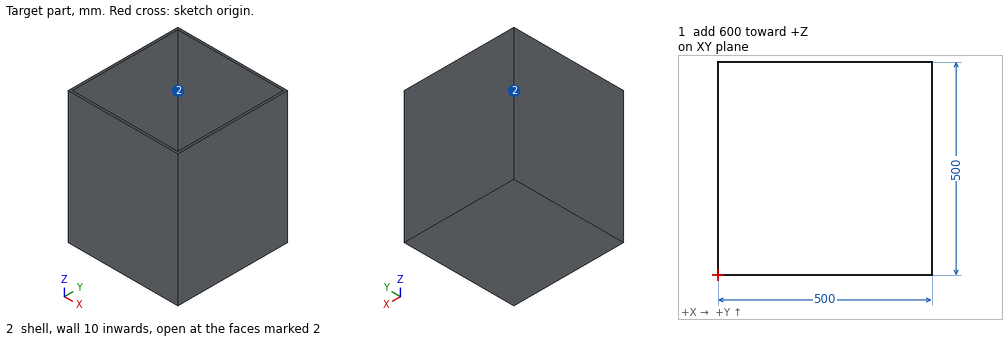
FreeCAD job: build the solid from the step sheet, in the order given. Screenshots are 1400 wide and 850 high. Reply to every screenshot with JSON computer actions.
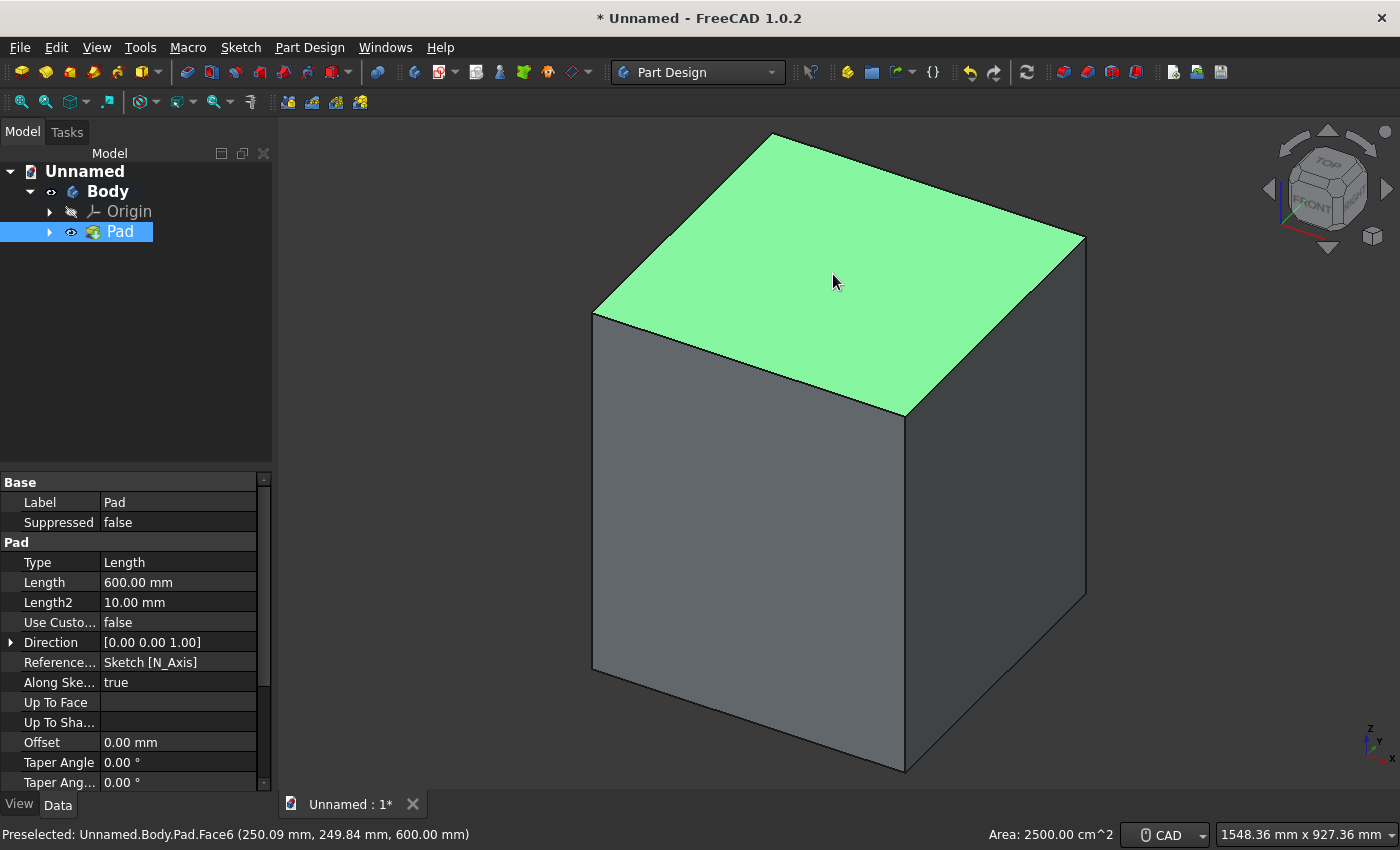
{"action": "left_click", "coordinate": [1136, 72]}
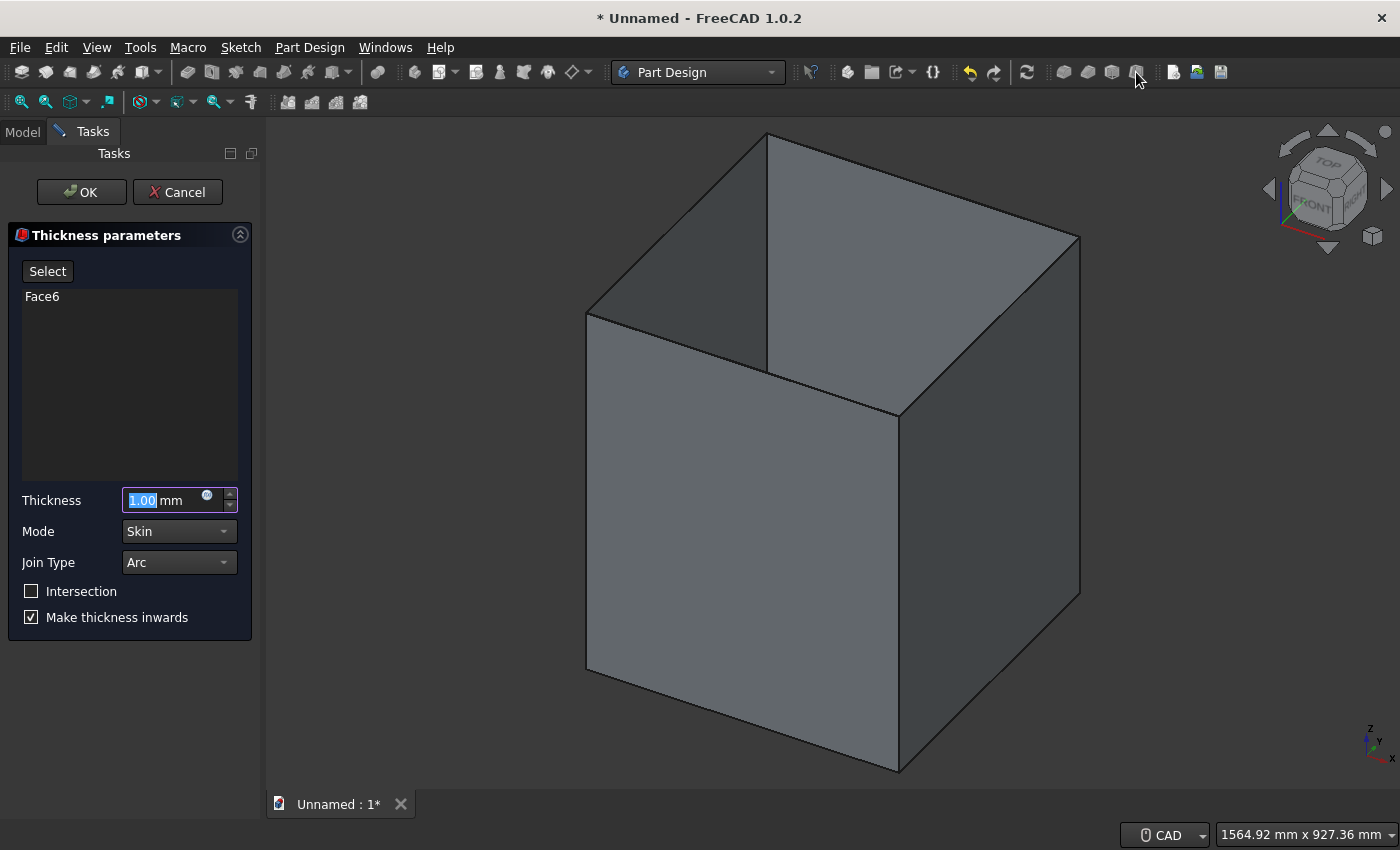
{"action": "type", "text": "10"}
{"action": "key", "text": "Tab"}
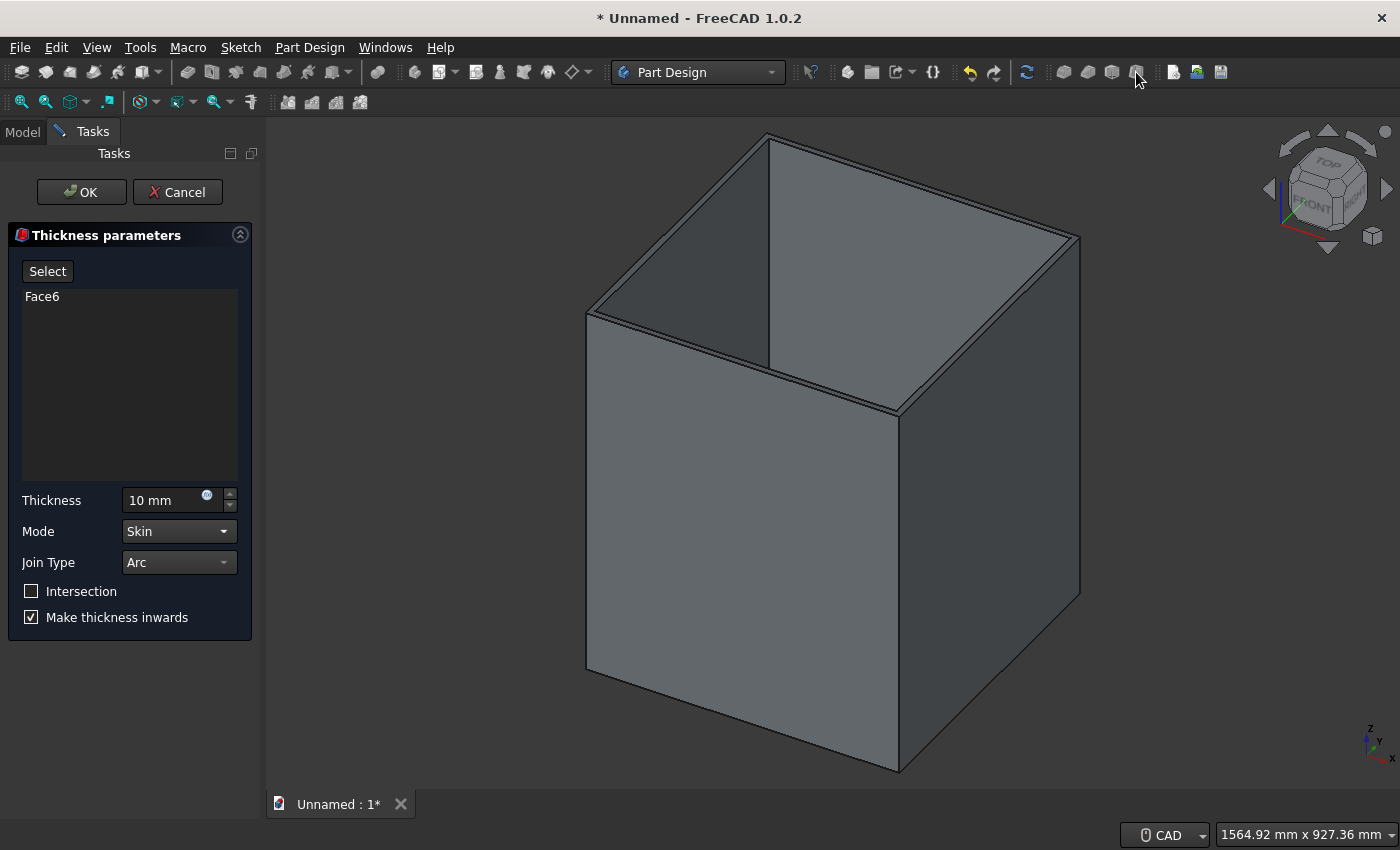
{"action": "left_click", "coordinate": [180, 562]}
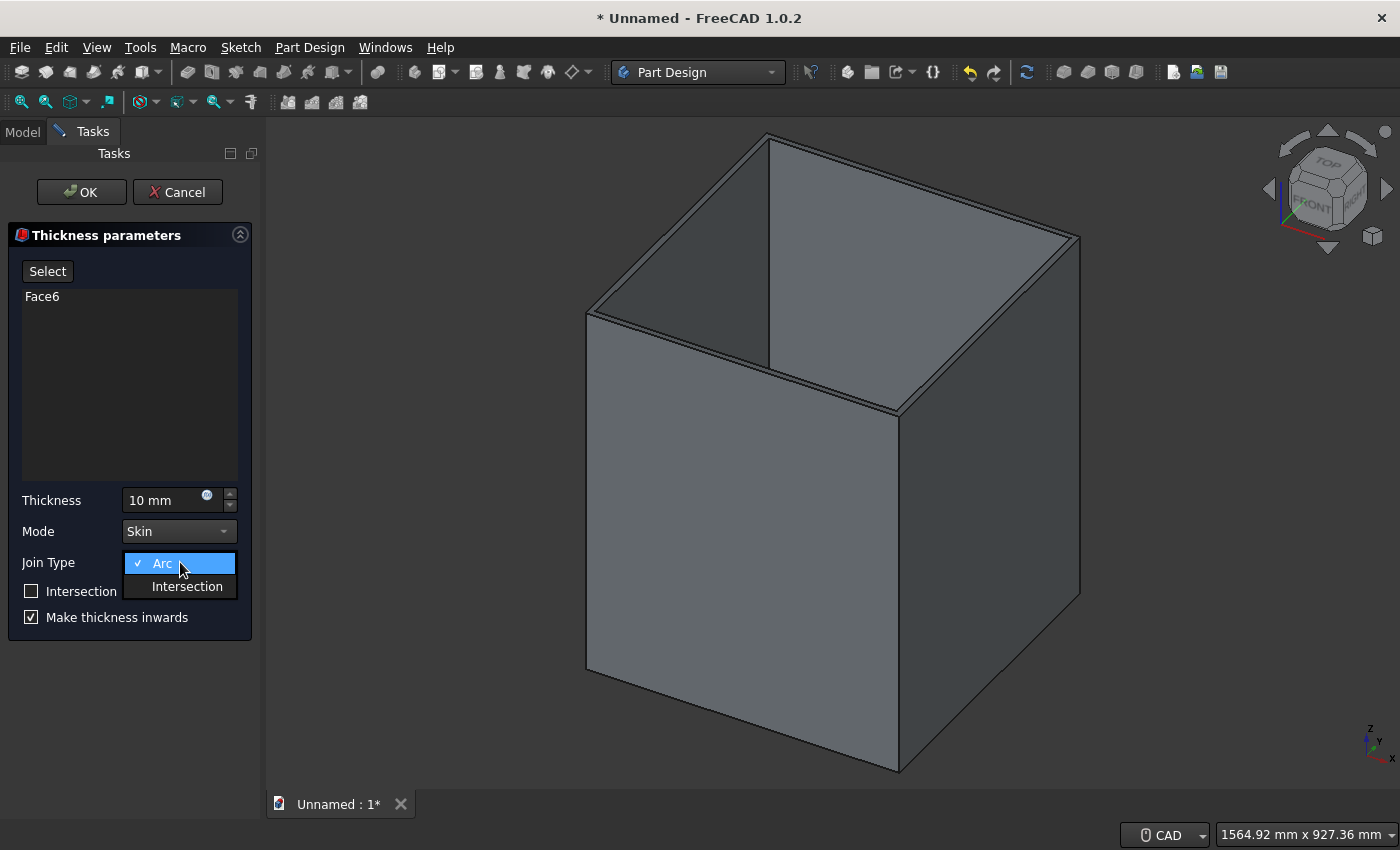
{"action": "left_click", "coordinate": [179, 586]}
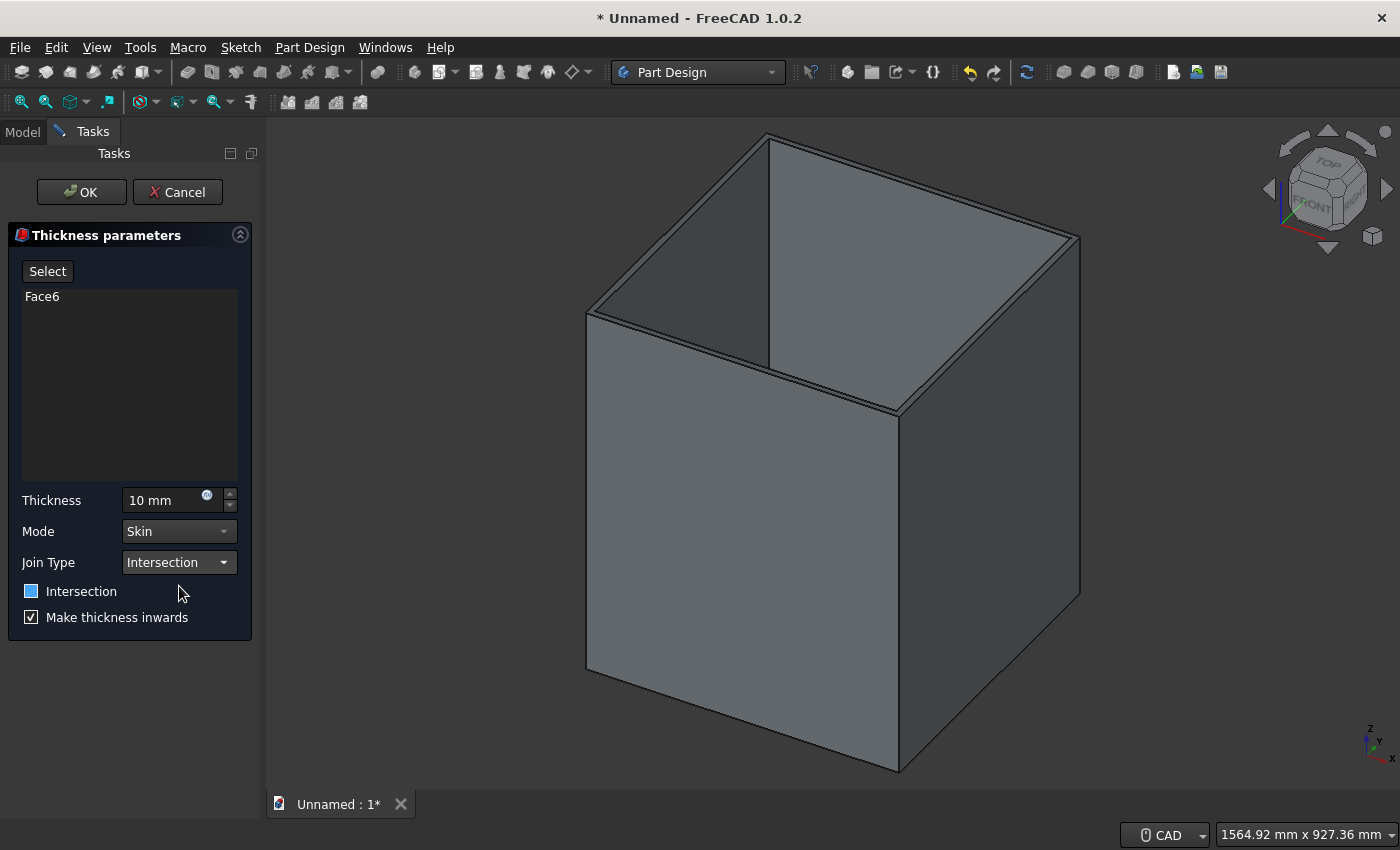
{"action": "left_click", "coordinate": [82, 192]}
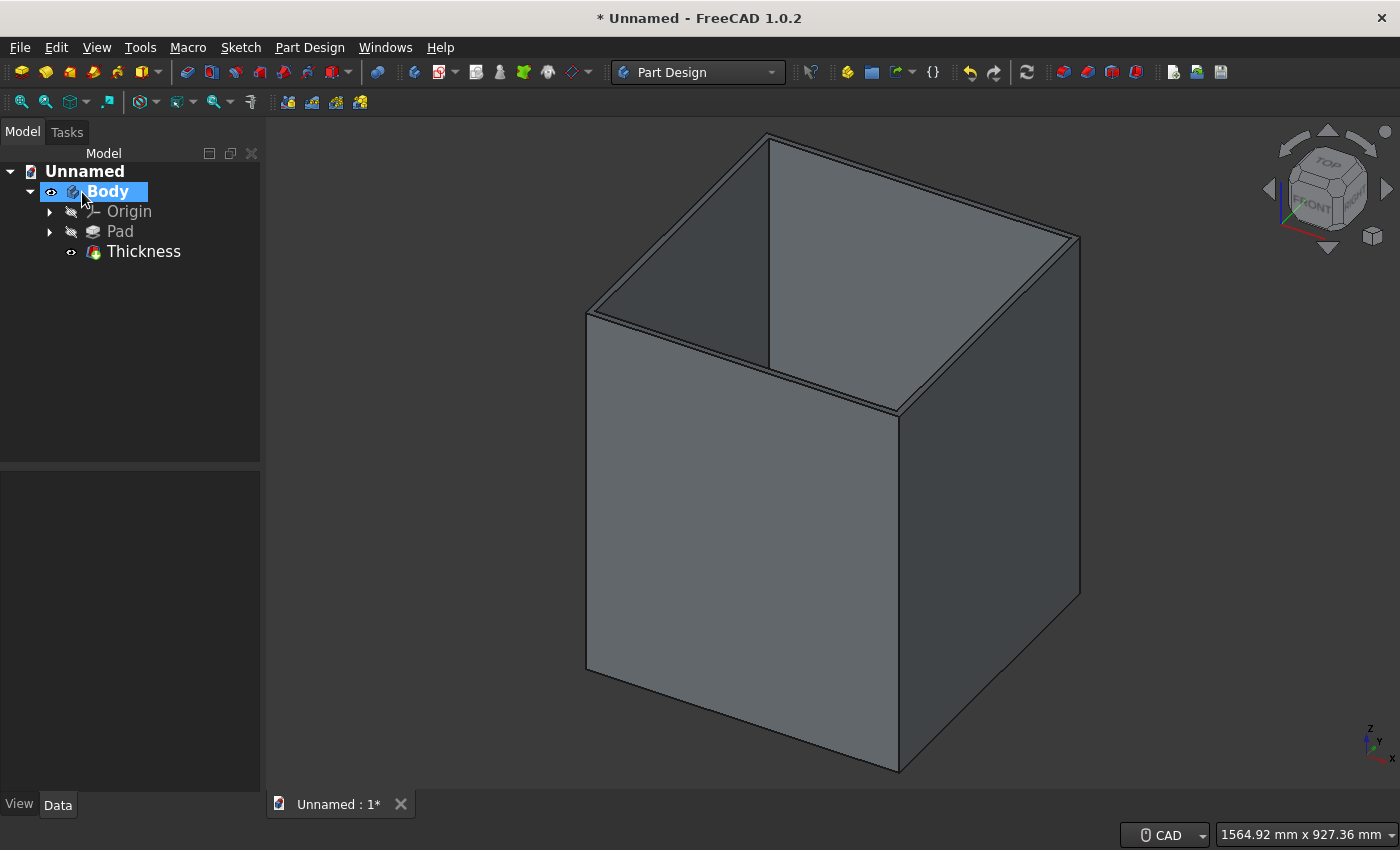
{"action": "key", "text": "0"}